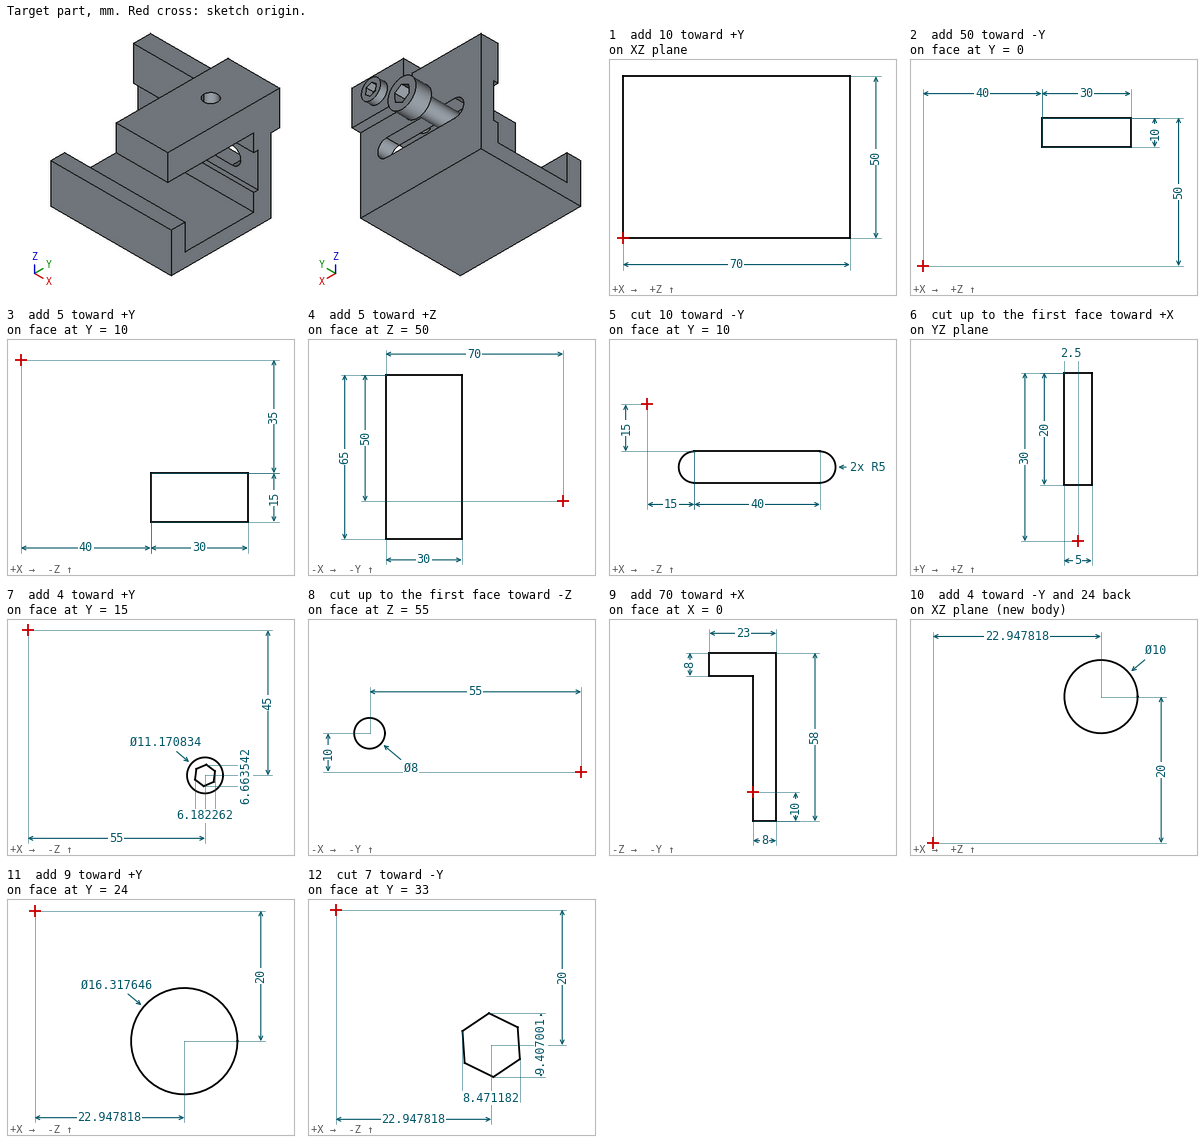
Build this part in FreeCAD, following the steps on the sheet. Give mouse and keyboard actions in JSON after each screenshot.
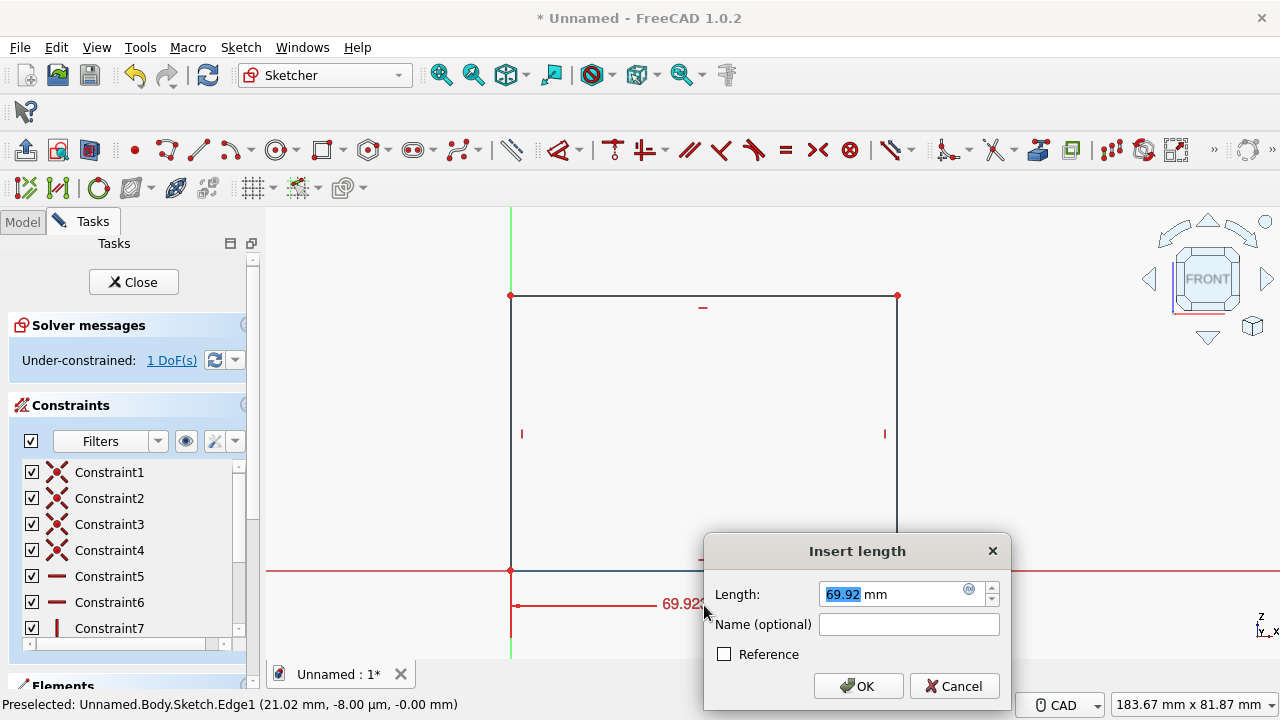
{"action": "type", "text": "70"}
{"action": "key", "text": "Return"}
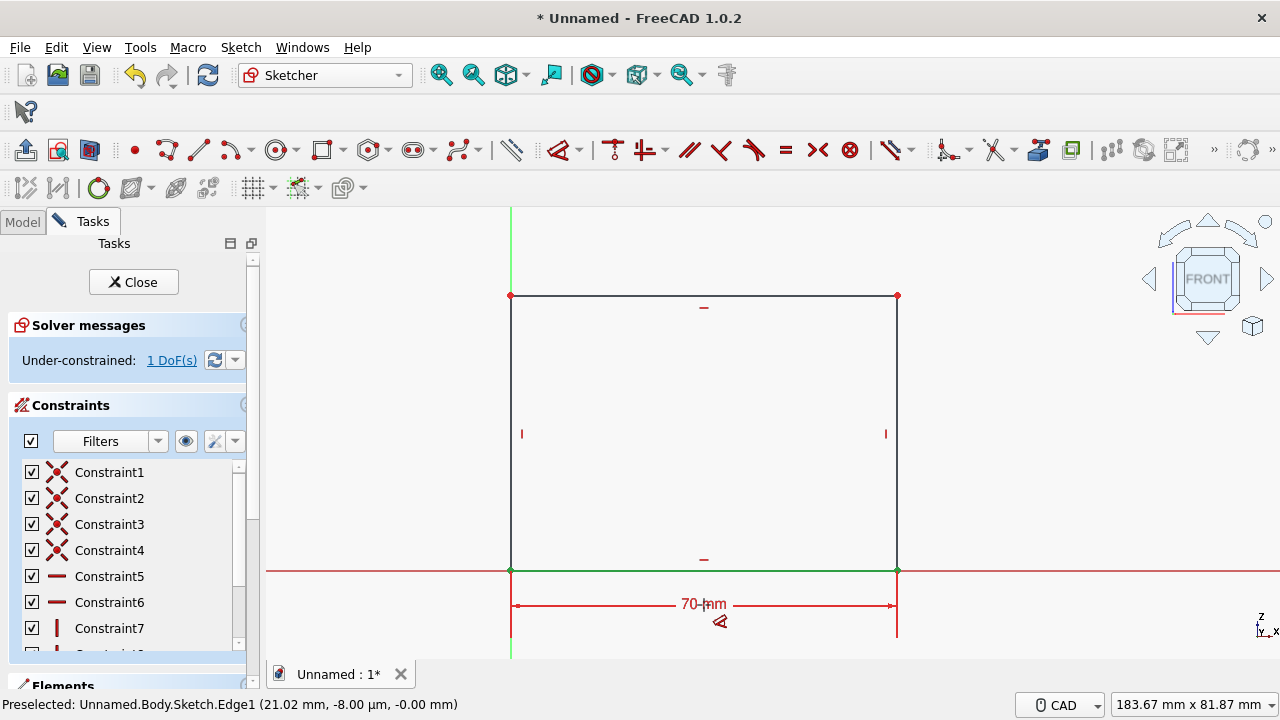
{"action": "left_click", "coordinate": [897, 488]}
{"action": "left_click", "coordinate": [931, 433]}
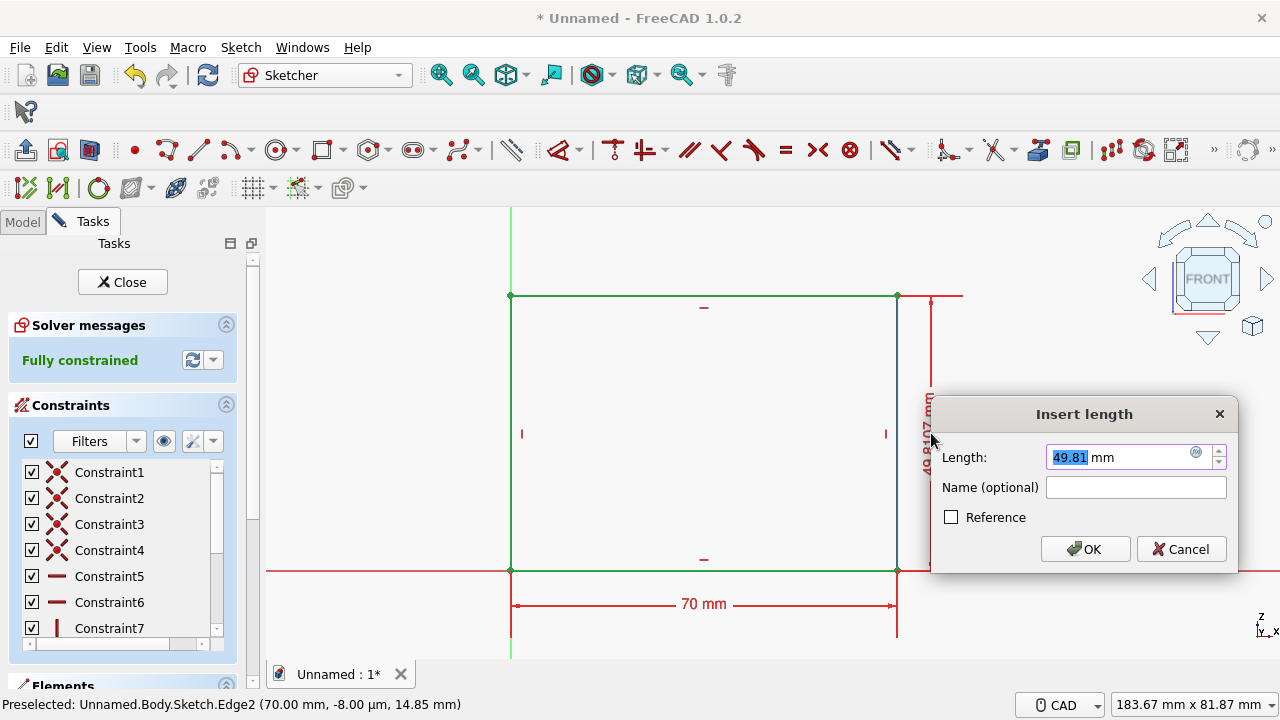
{"action": "type", "text": "50"}
{"action": "key", "text": "Return"}
{"action": "key", "text": "Escape"}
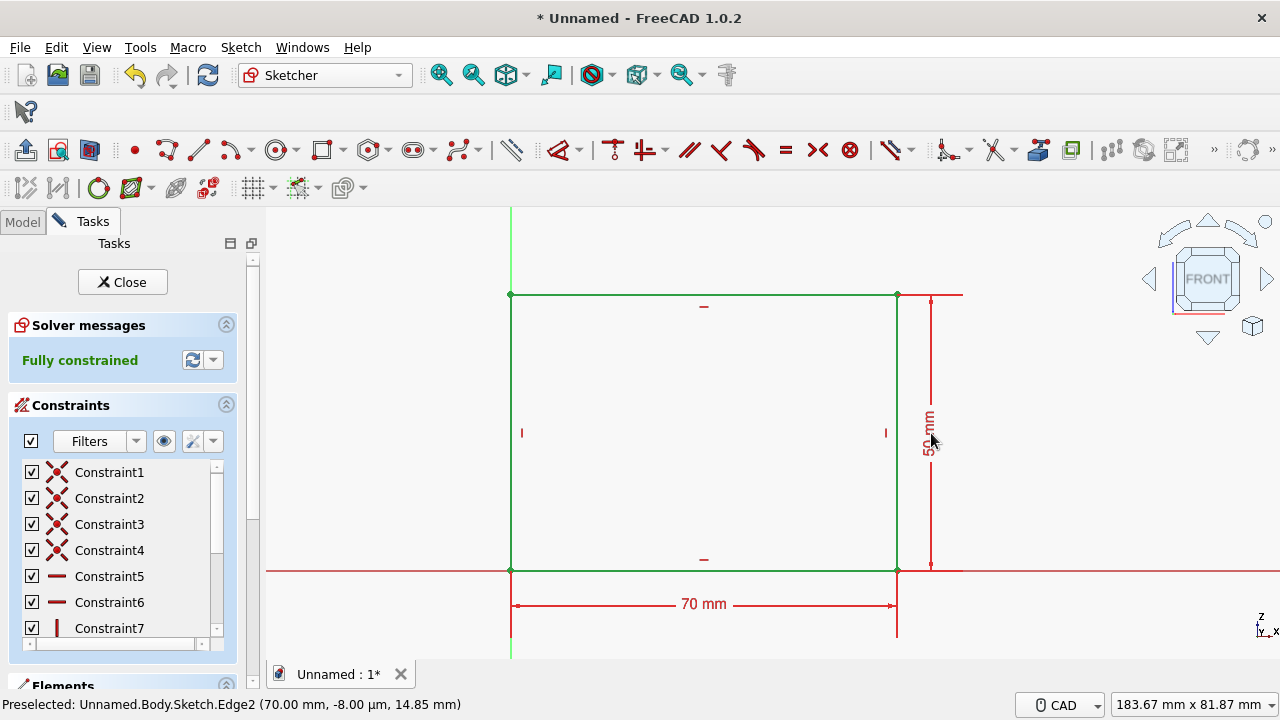
{"action": "left_click", "coordinate": [123, 282]}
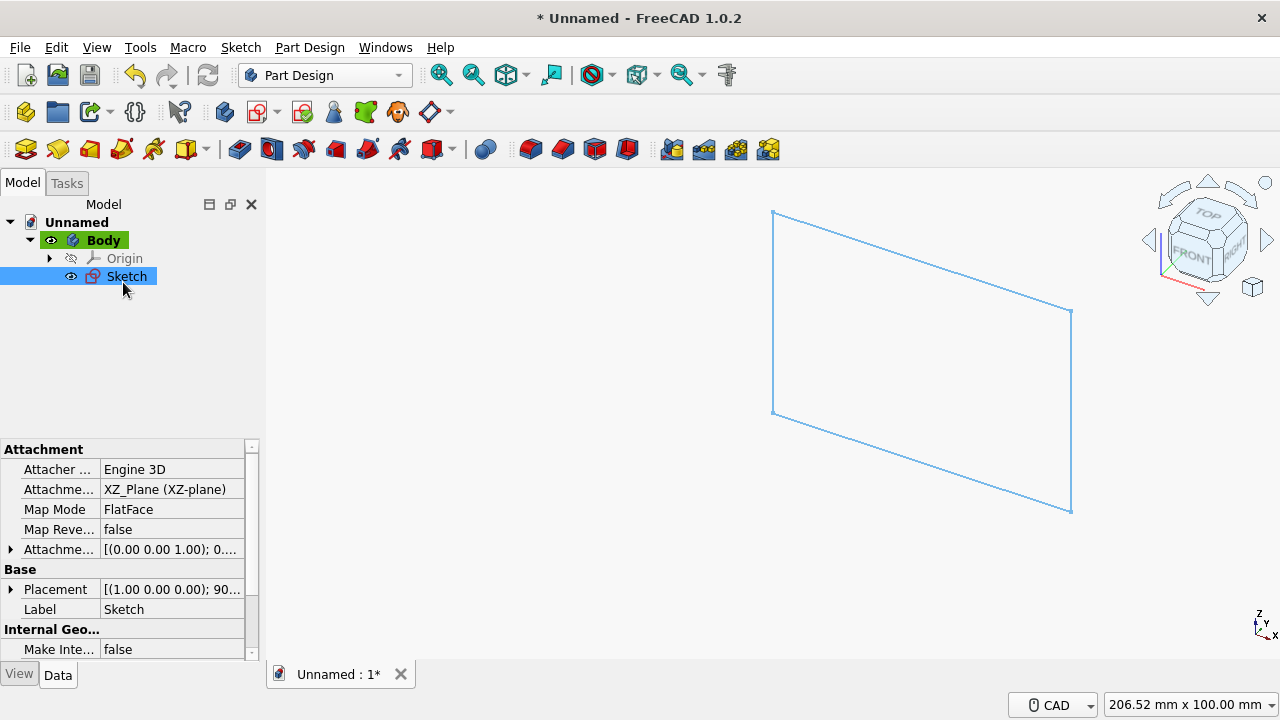
{"action": "left_click", "coordinate": [26, 150]}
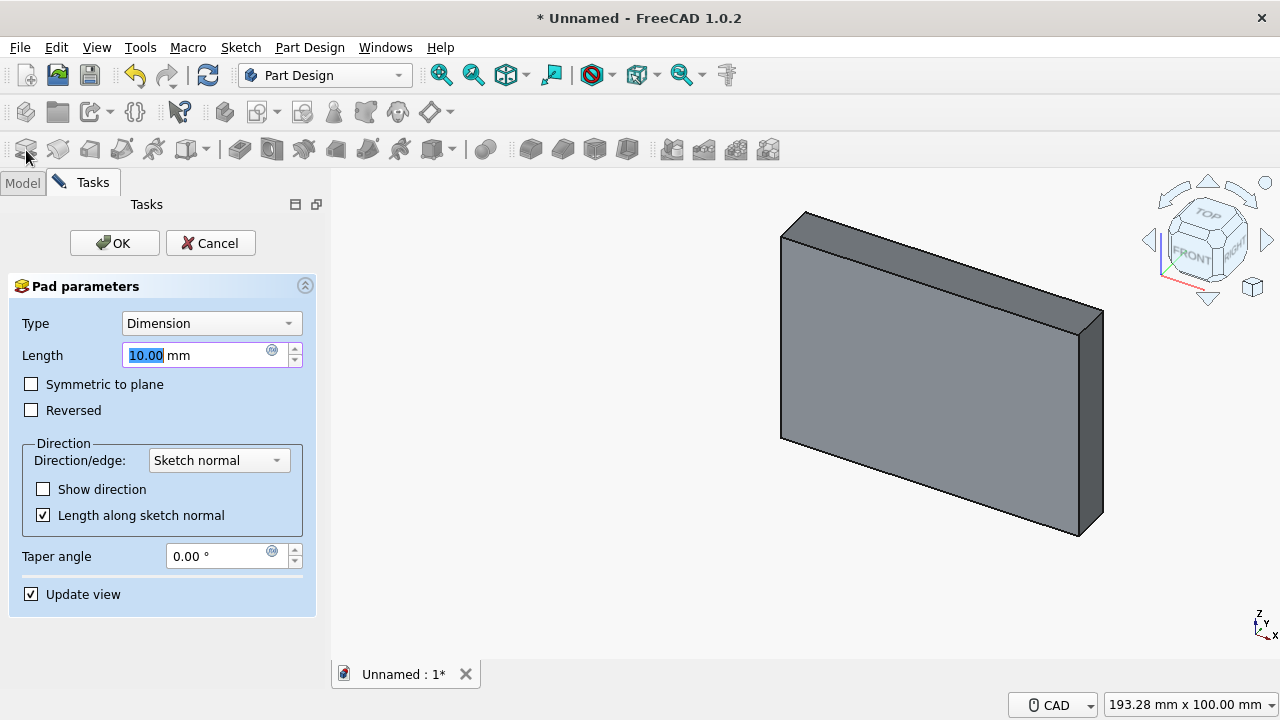
{"action": "type", "text": "10"}
{"action": "key", "text": "Tab"}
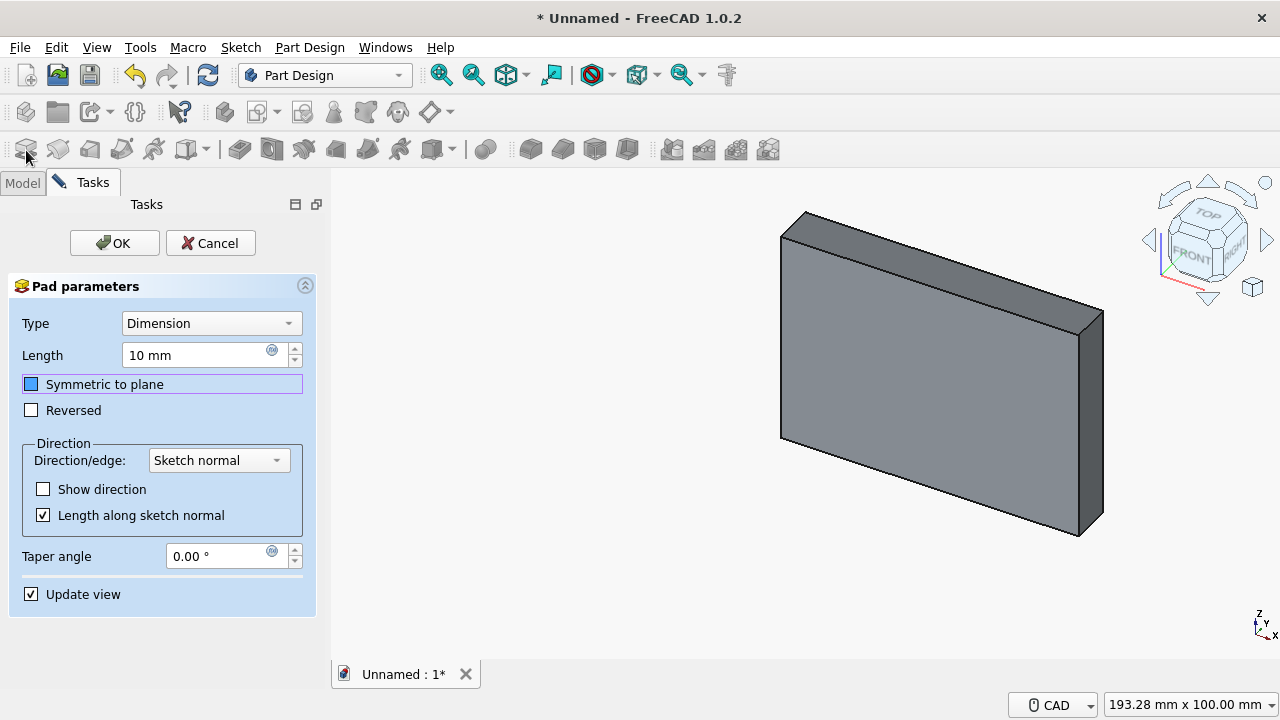
{"action": "left_click", "coordinate": [30, 410]}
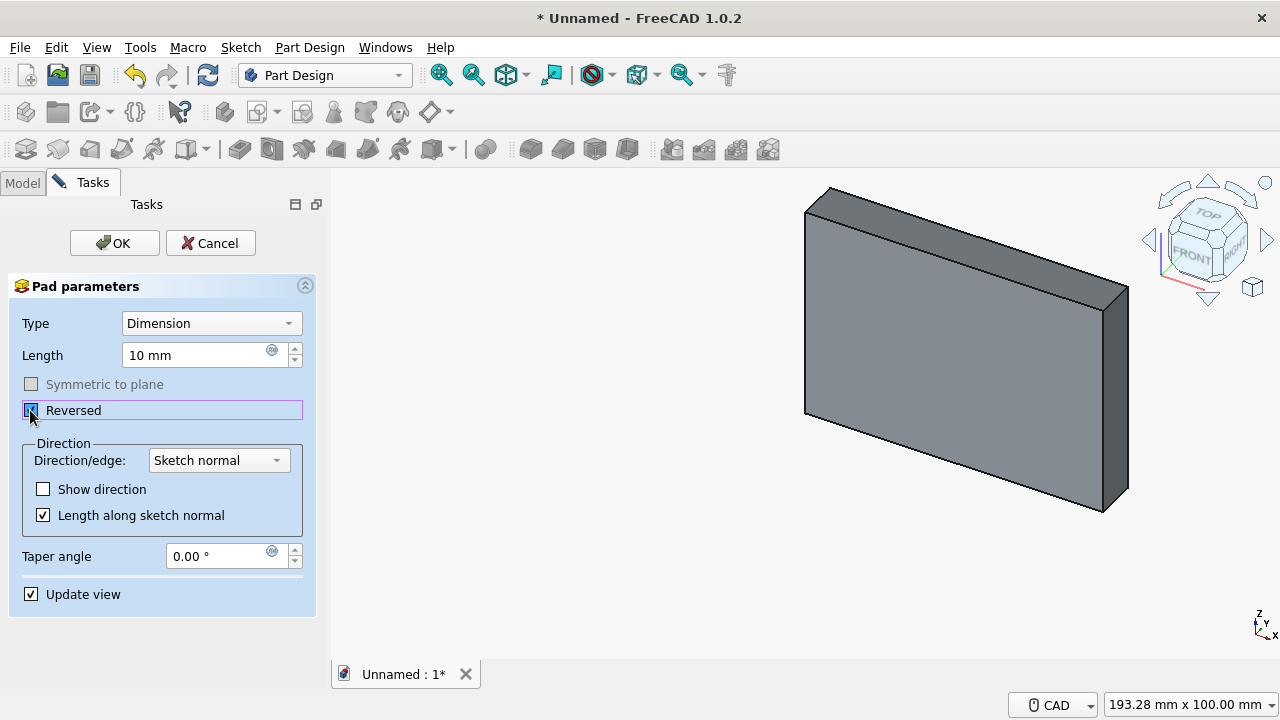
{"action": "left_click", "coordinate": [115, 243]}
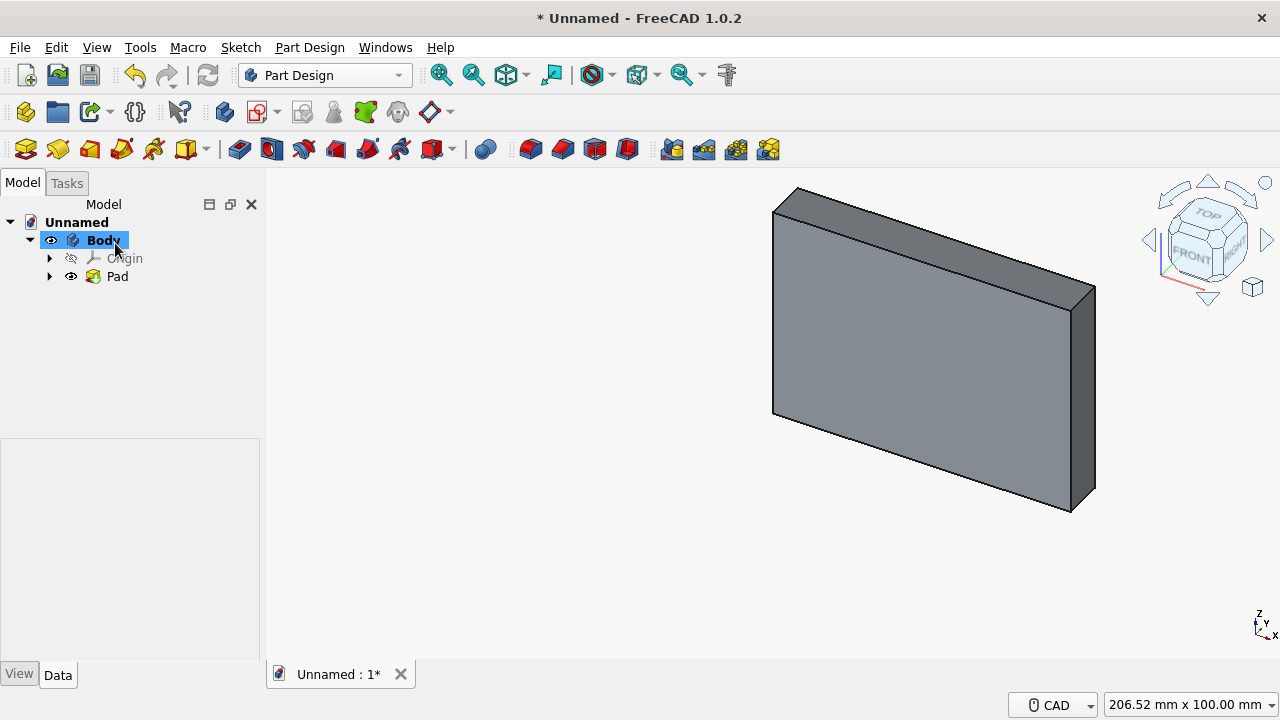
{"action": "left_click", "coordinate": [964, 375]}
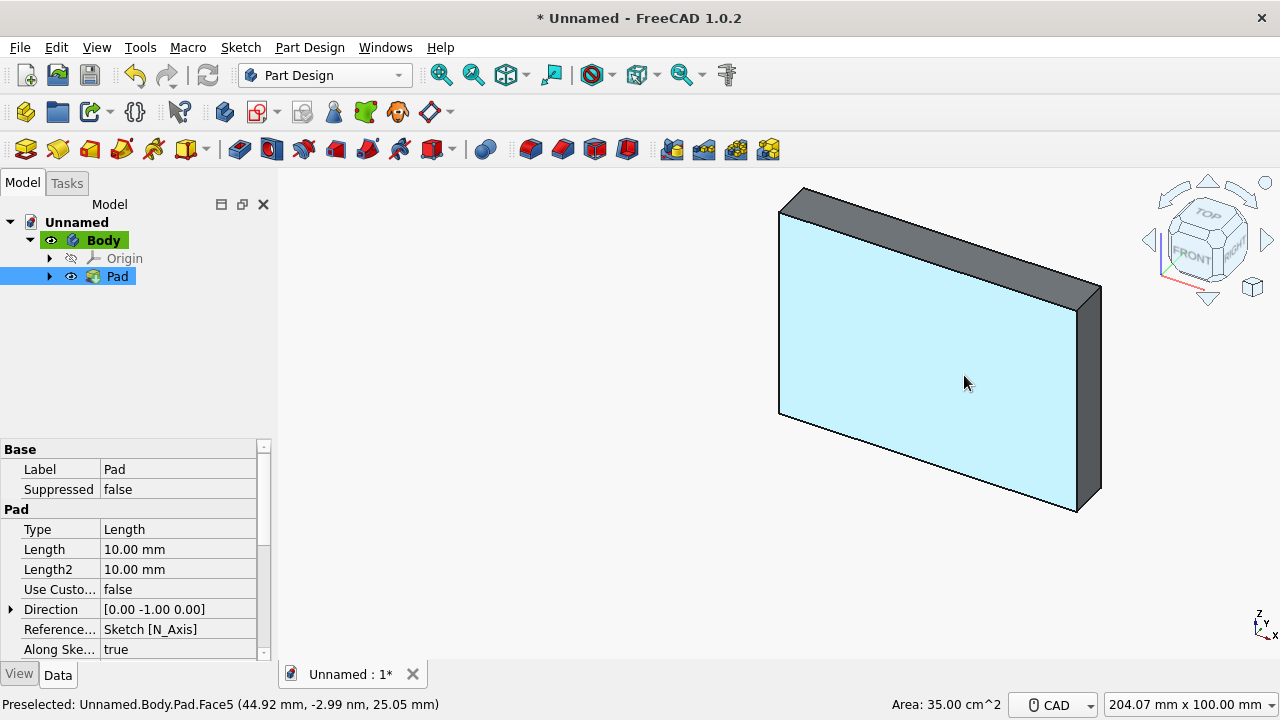
{"action": "left_click", "coordinate": [258, 112]}